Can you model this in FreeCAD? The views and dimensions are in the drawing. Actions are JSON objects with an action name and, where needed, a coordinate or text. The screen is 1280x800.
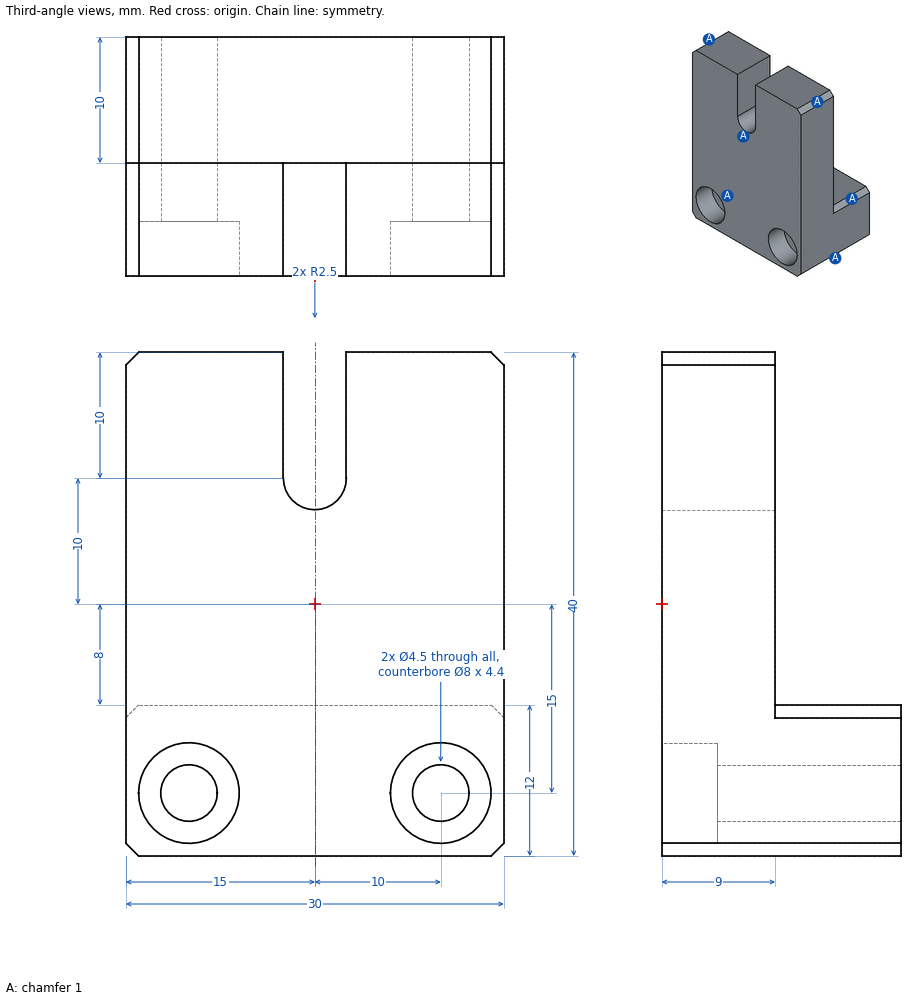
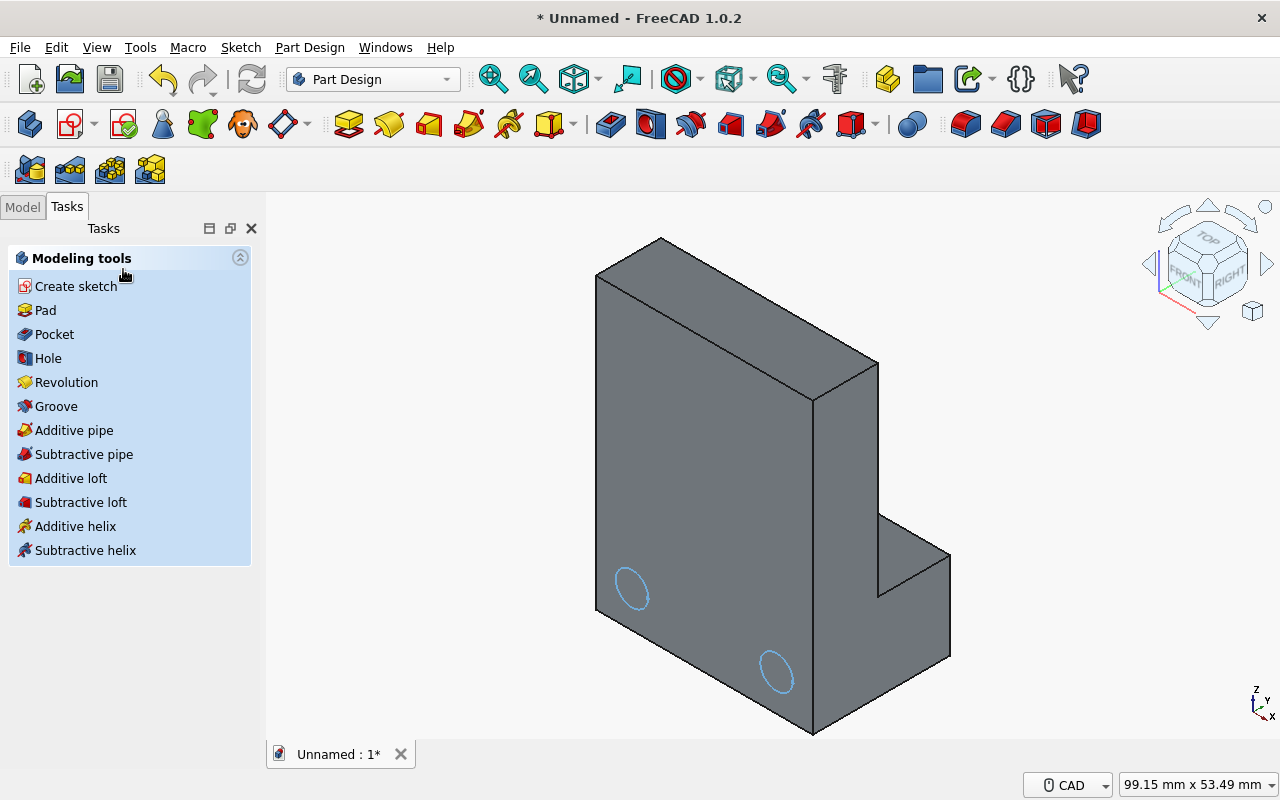
{"action": "left_click", "coordinate": [652, 124]}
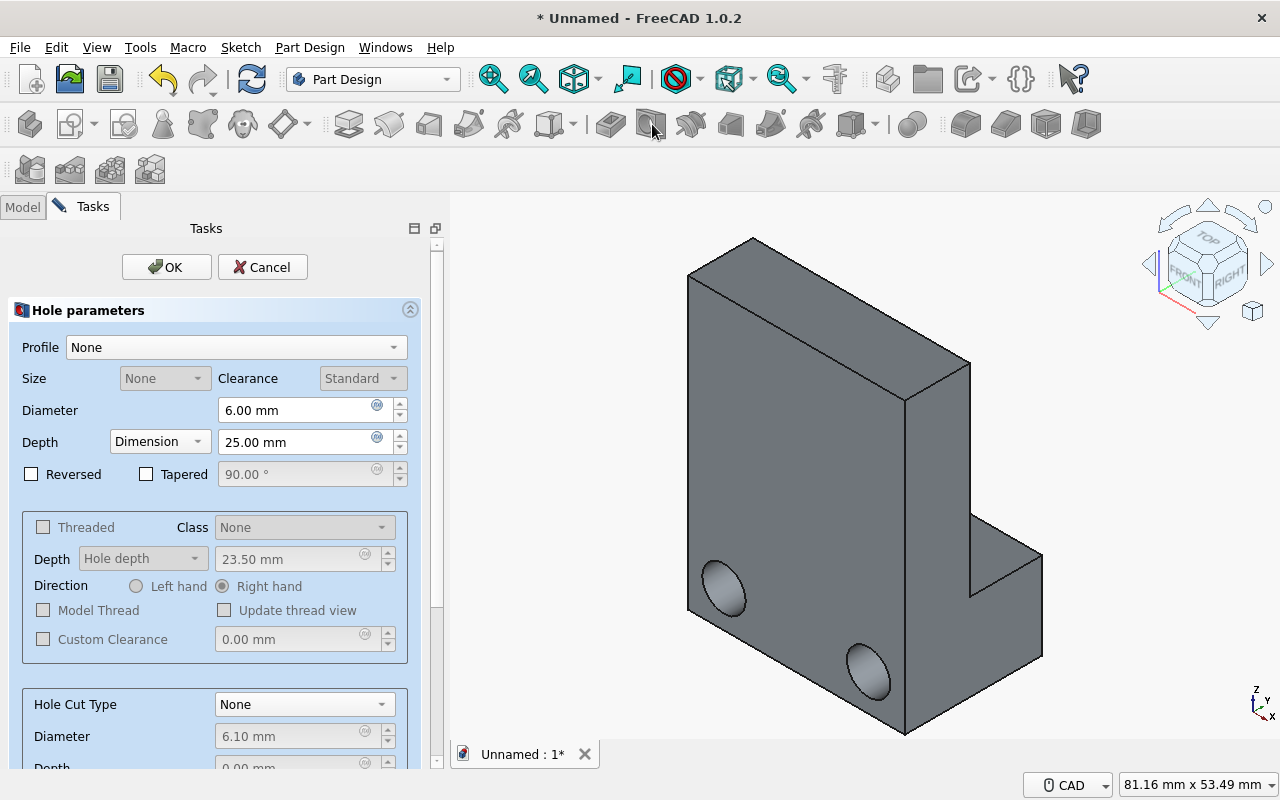
{"action": "triple_click", "coordinate": [305, 410]}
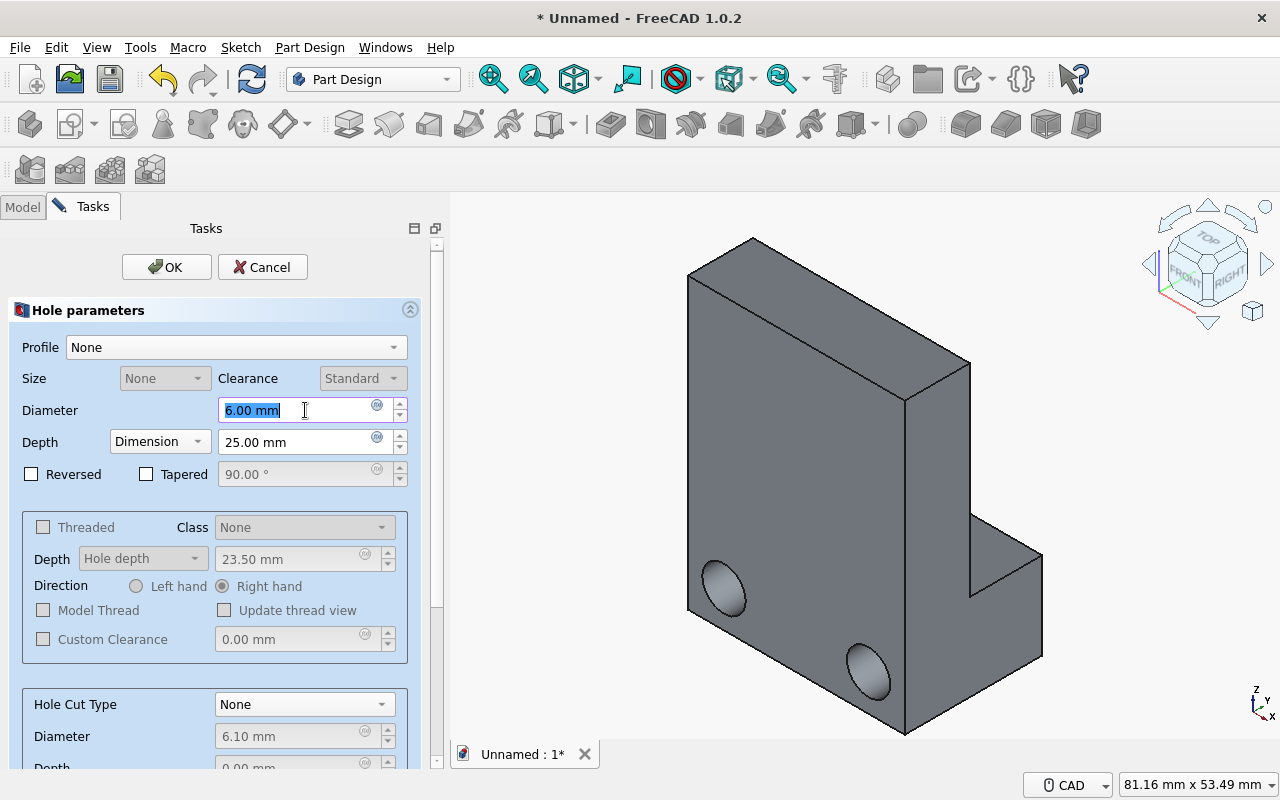
{"action": "type", "text": "4.5"}
{"action": "key", "text": "Tab"}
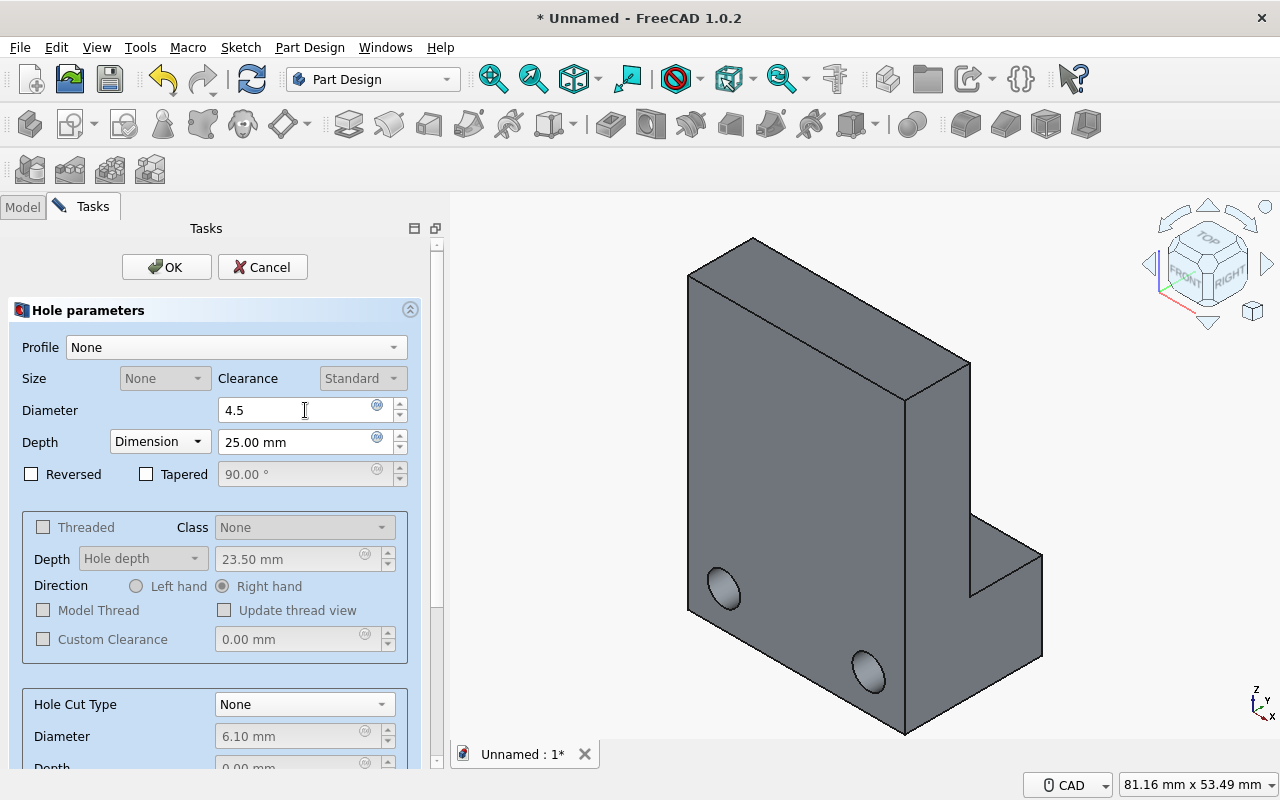
{"action": "left_click", "coordinate": [161, 442]}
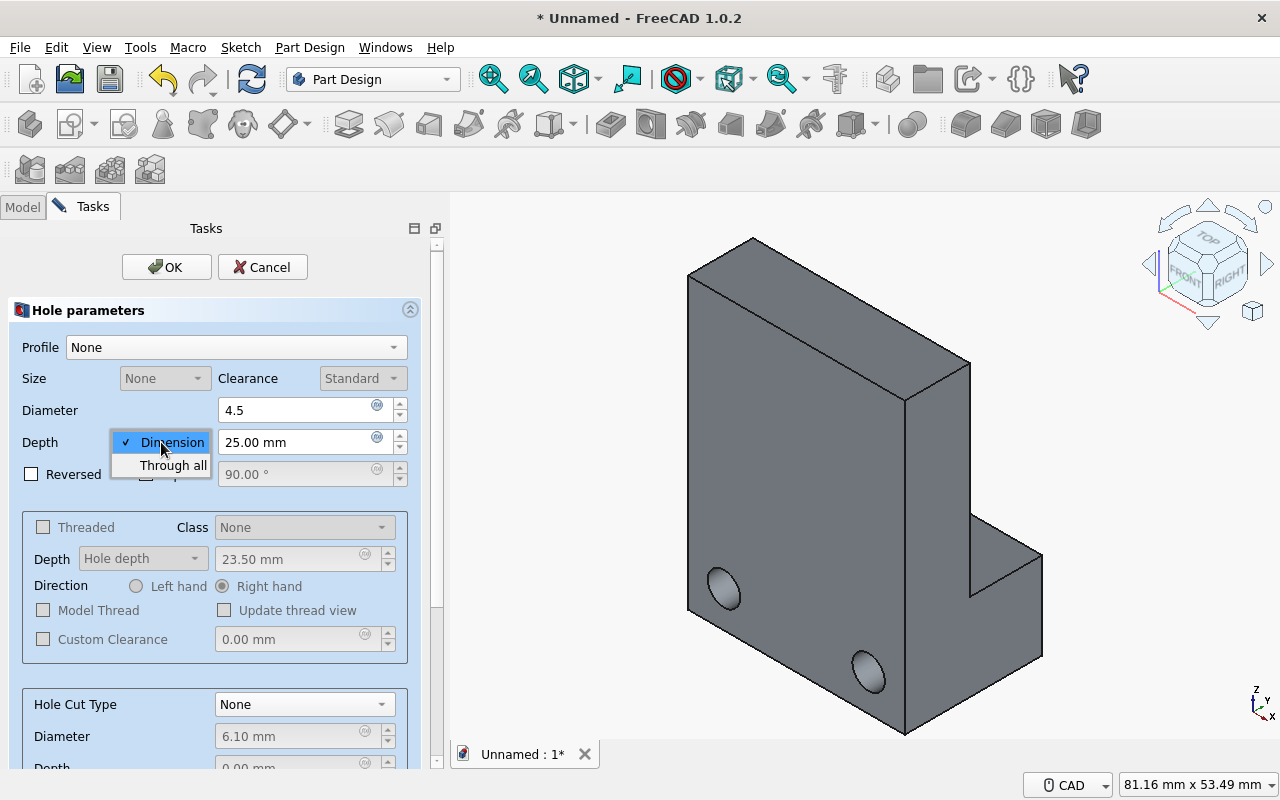
{"action": "left_click", "coordinate": [160, 466]}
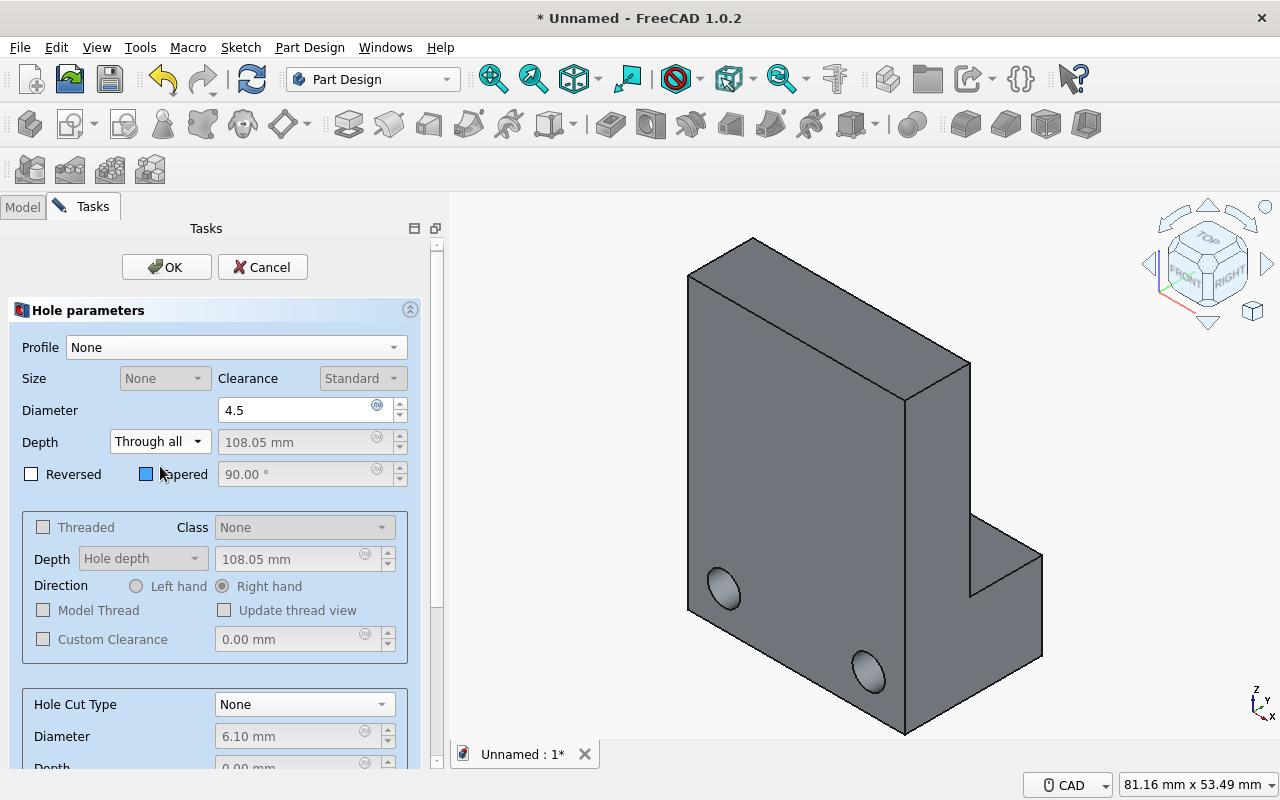
{"action": "left_click", "coordinate": [306, 704]}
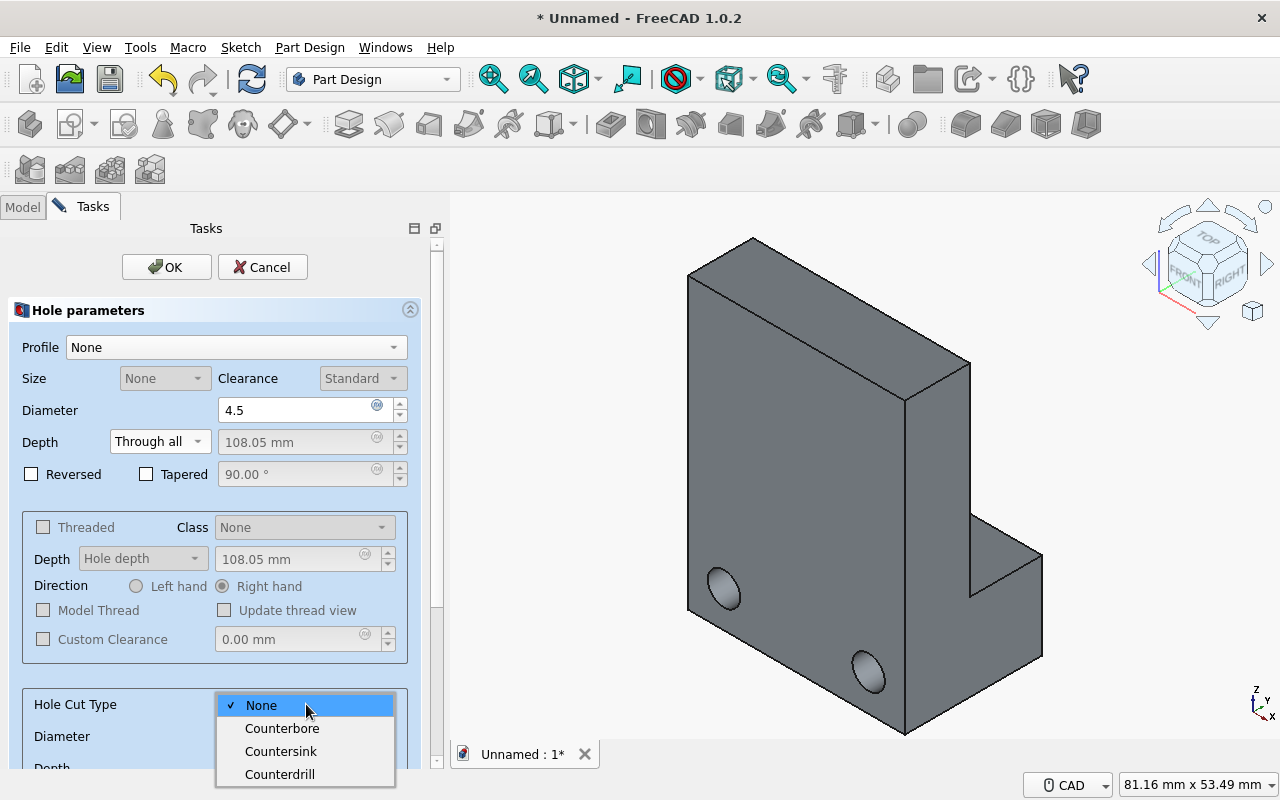
{"action": "left_click", "coordinate": [304, 728]}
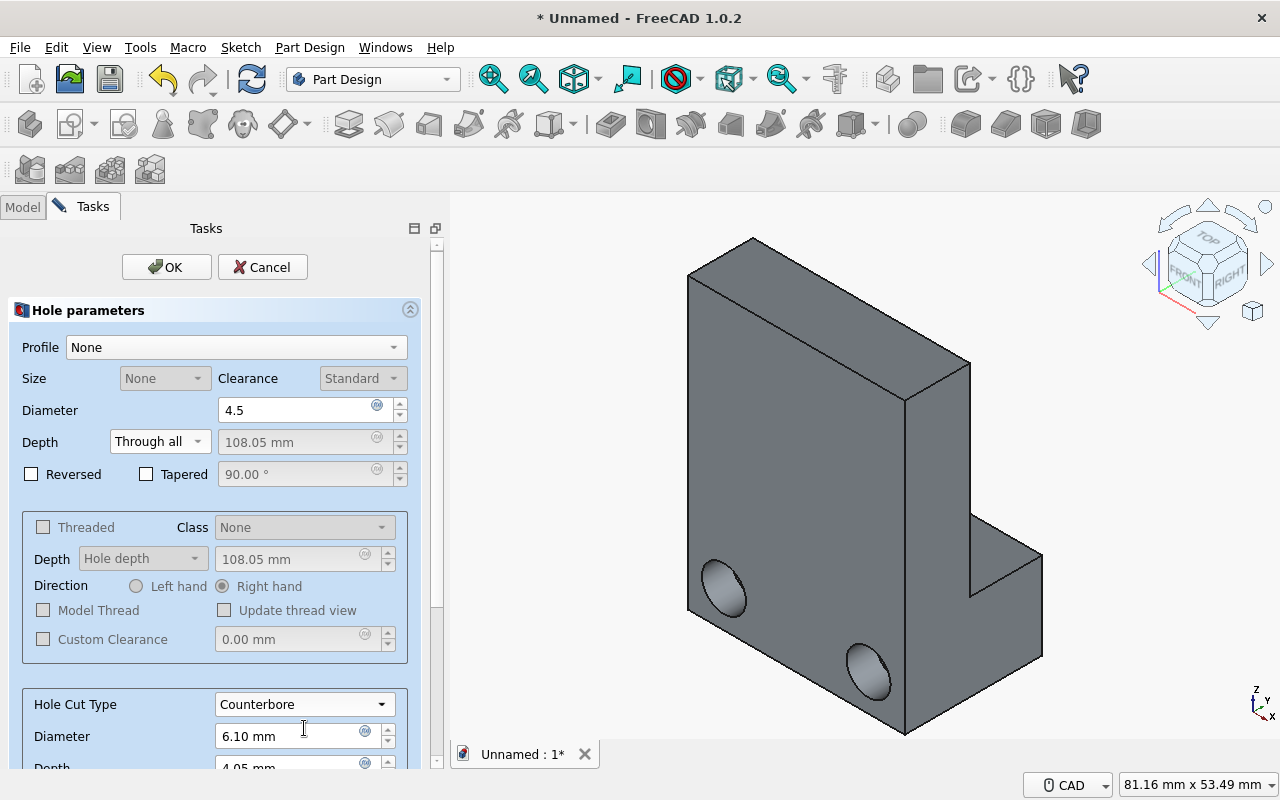
{"action": "triple_click", "coordinate": [298, 736]}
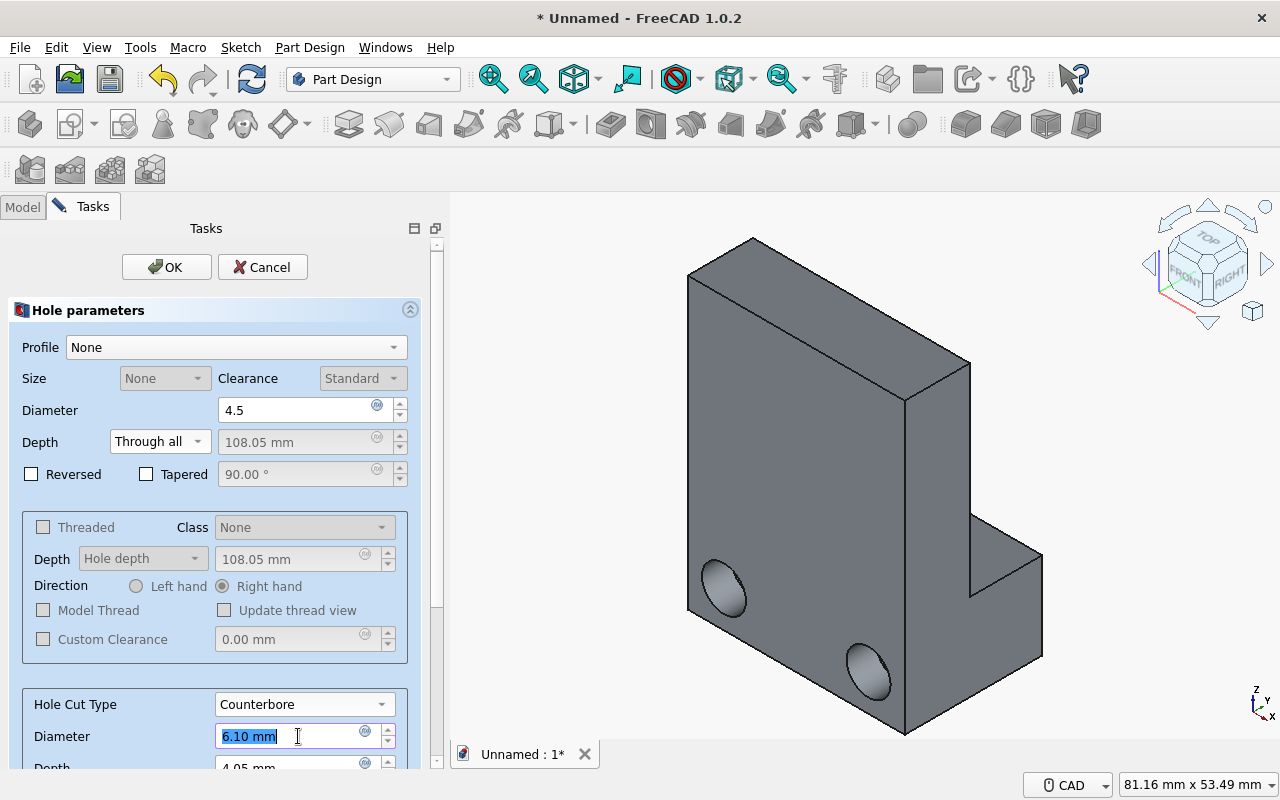
{"action": "type", "text": "8"}
{"action": "key", "text": "Tab"}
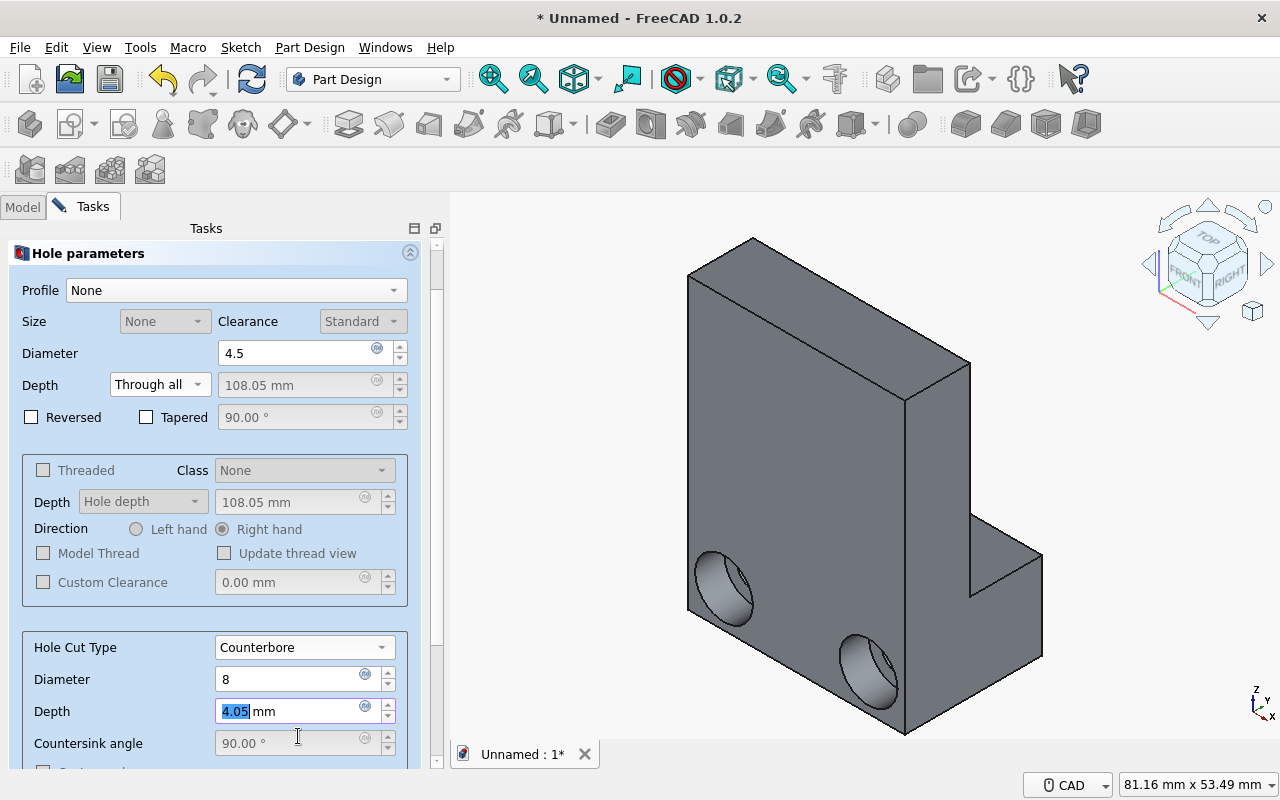
{"action": "type", "text": "4.4"}
{"action": "key", "text": "Tab"}